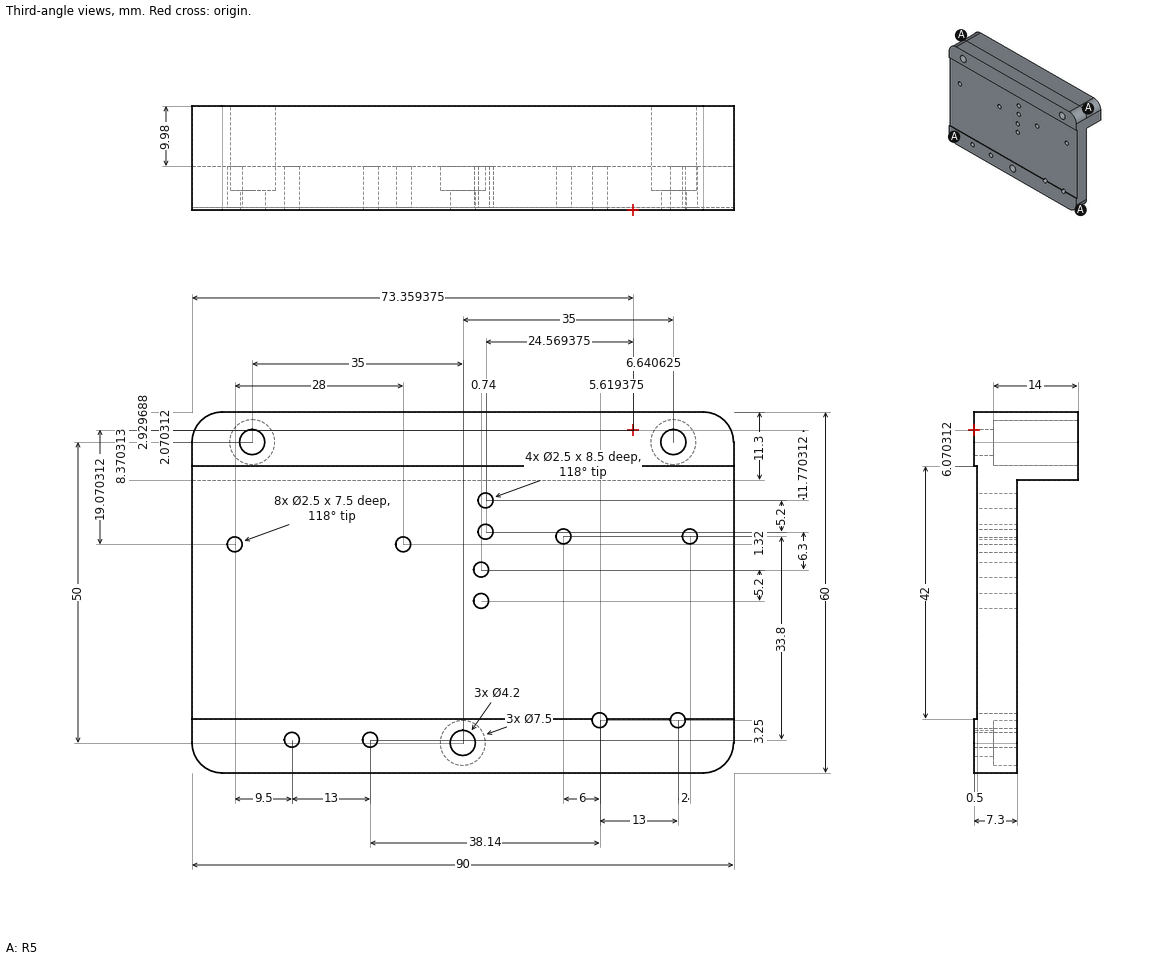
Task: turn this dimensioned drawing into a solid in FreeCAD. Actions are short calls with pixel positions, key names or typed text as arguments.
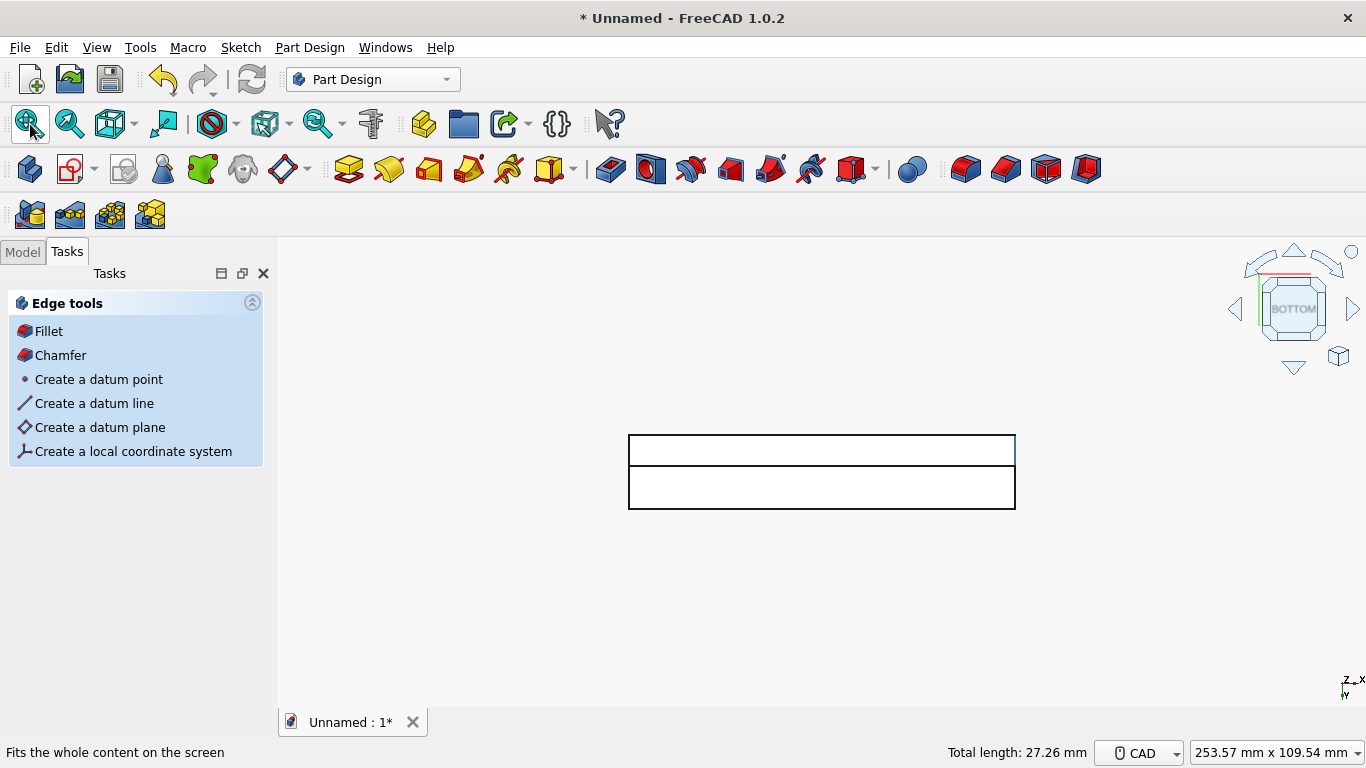
click(629, 450, ctrl)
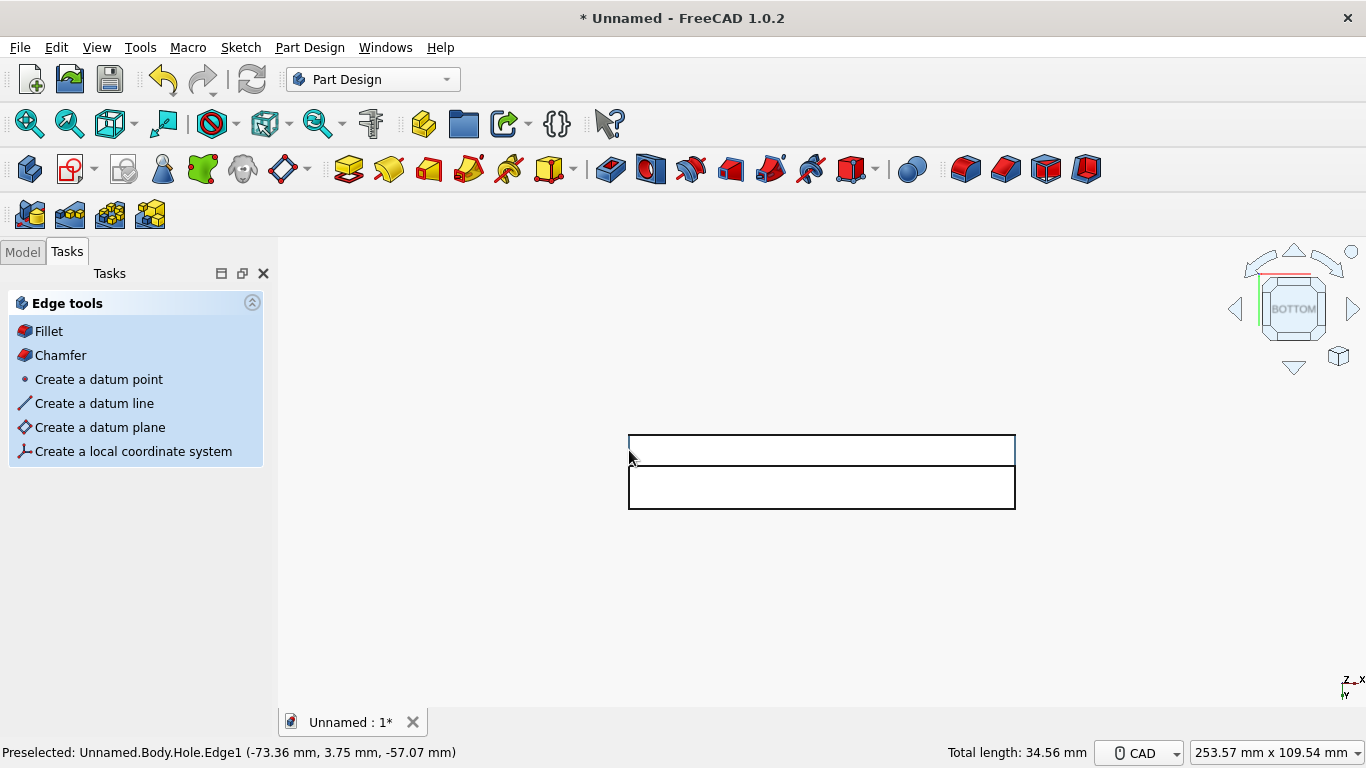
click(966, 170)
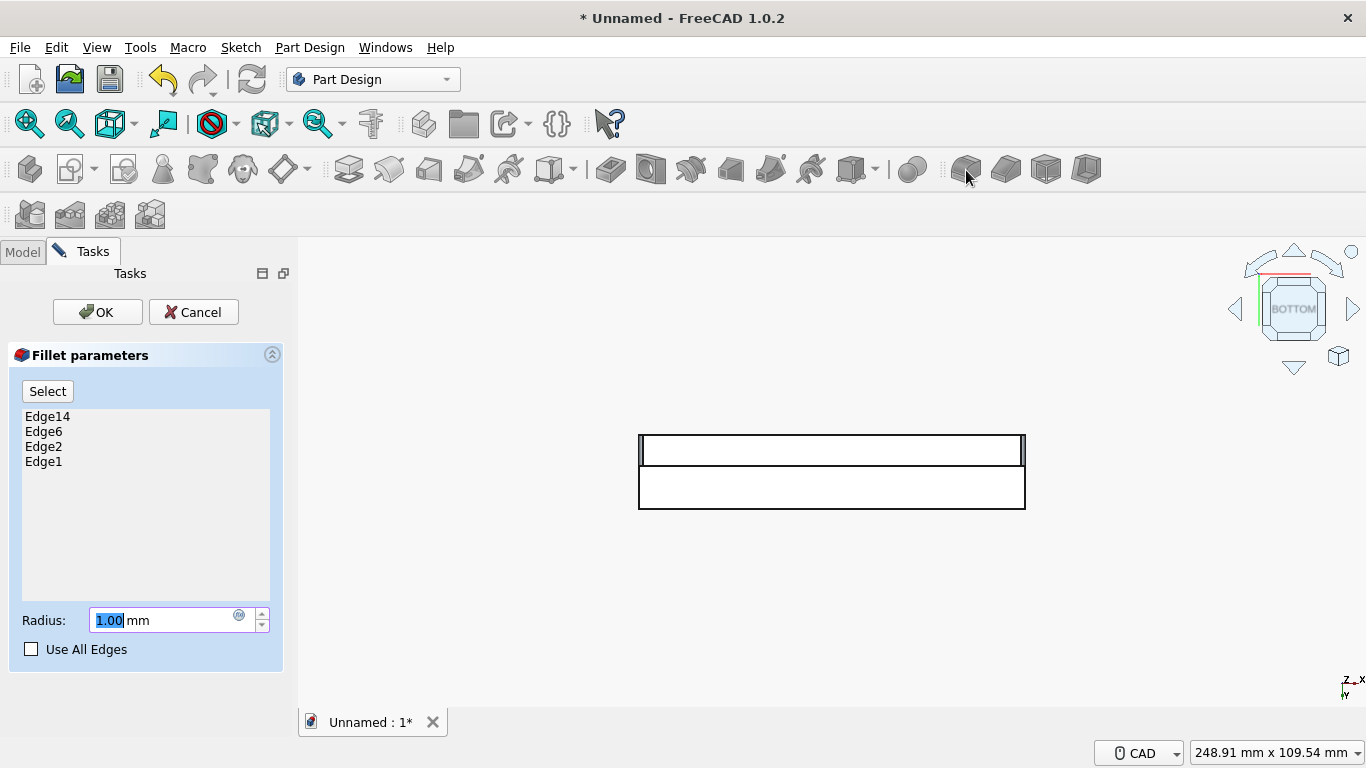
text(5)
key(Tab)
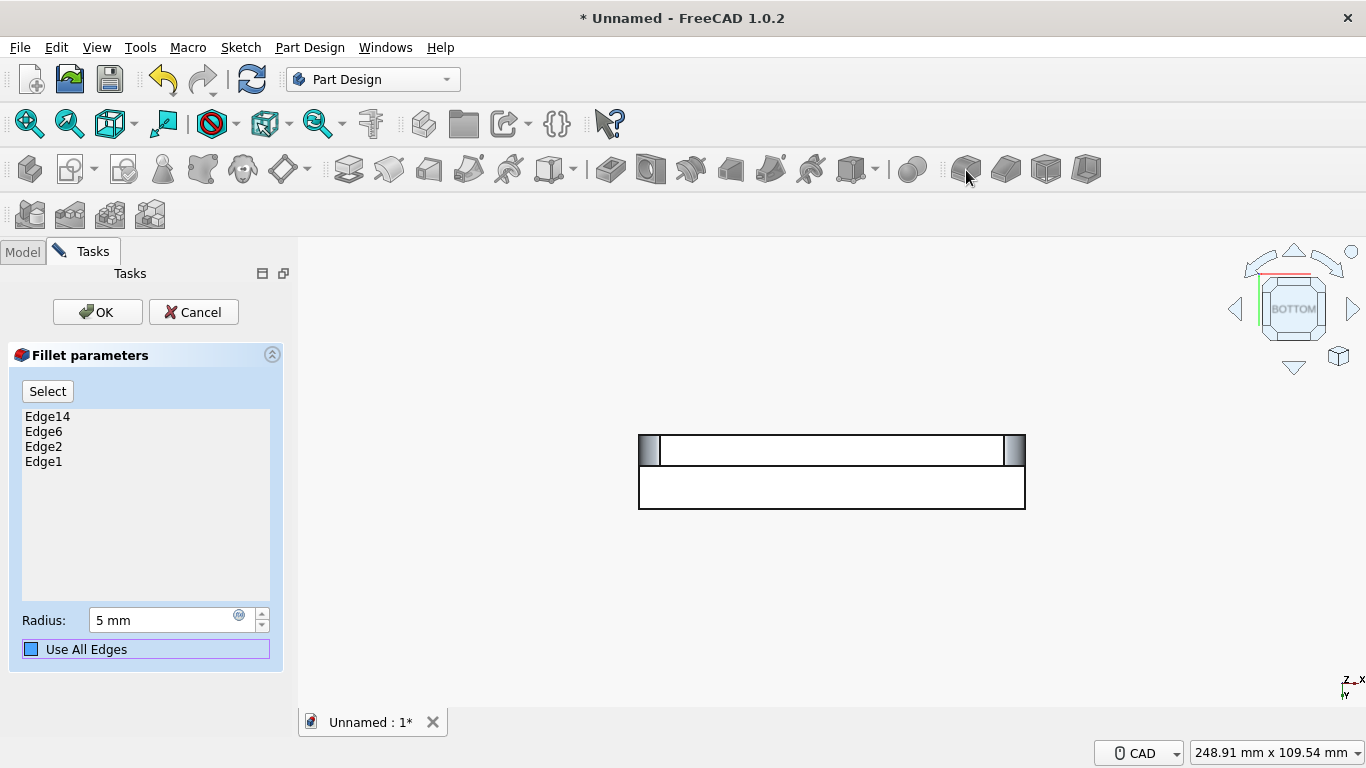
click(98, 312)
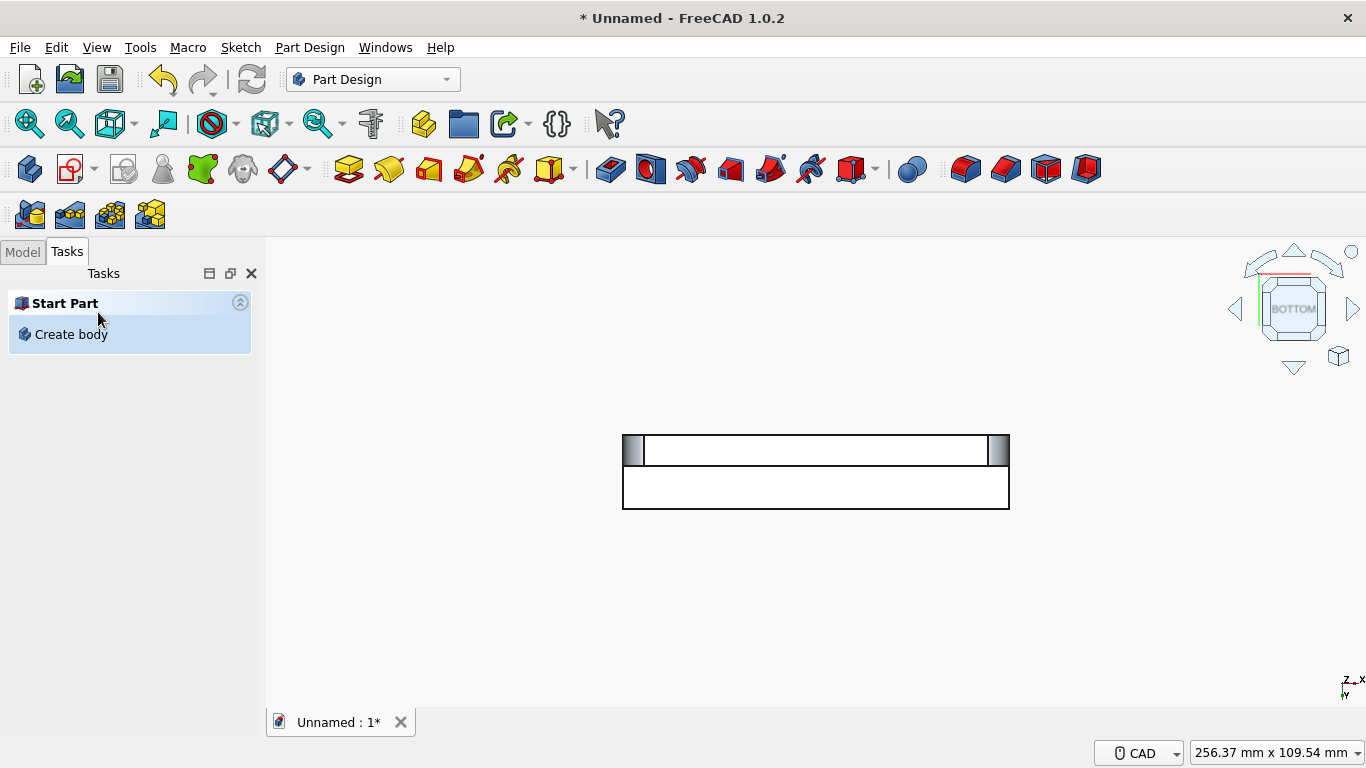
click(30, 124)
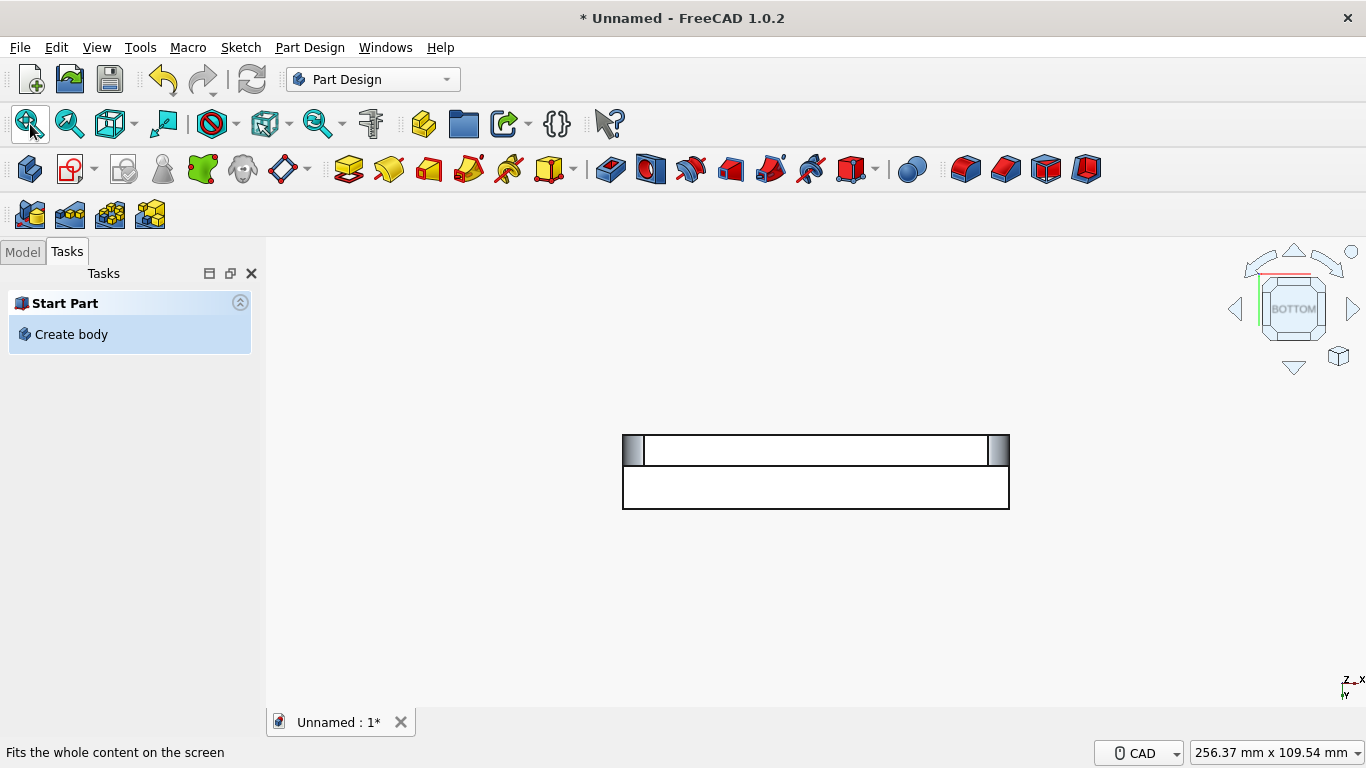
key(4)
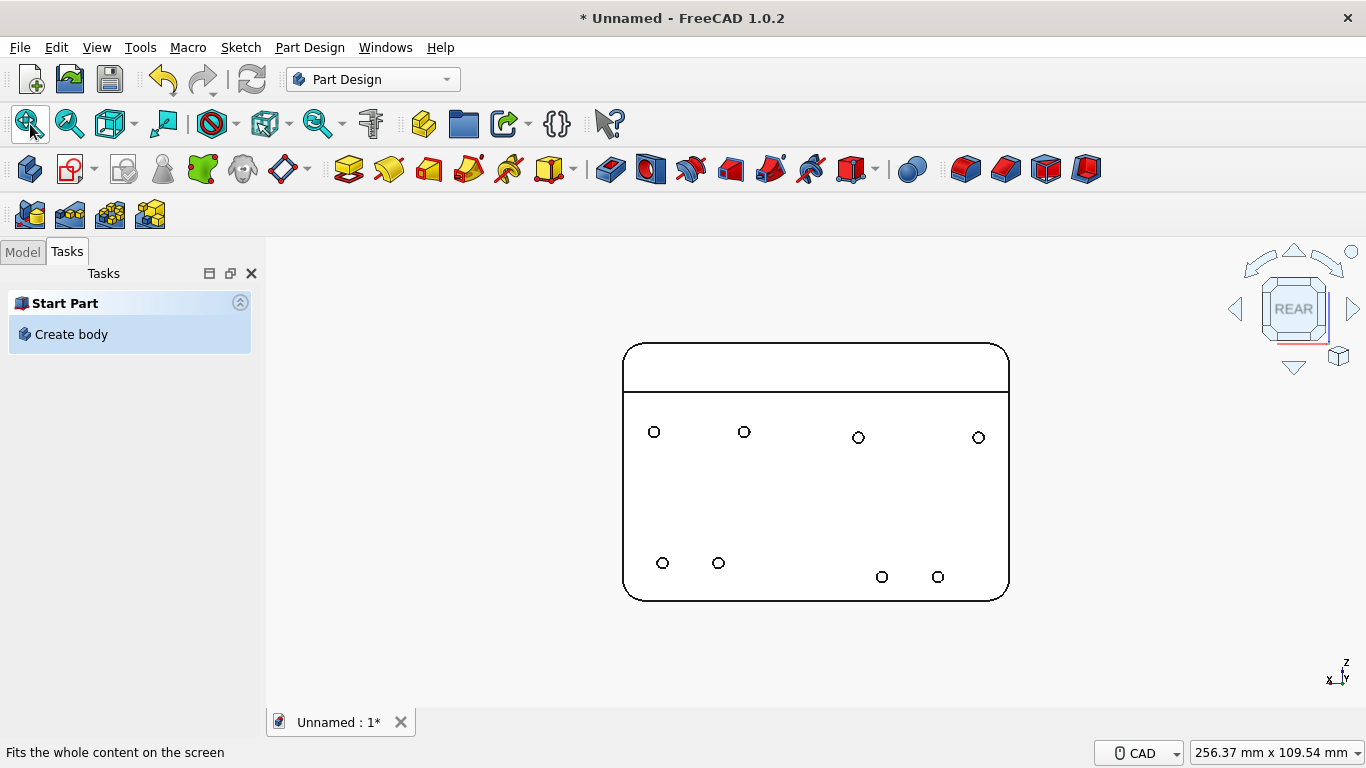
click(650, 367)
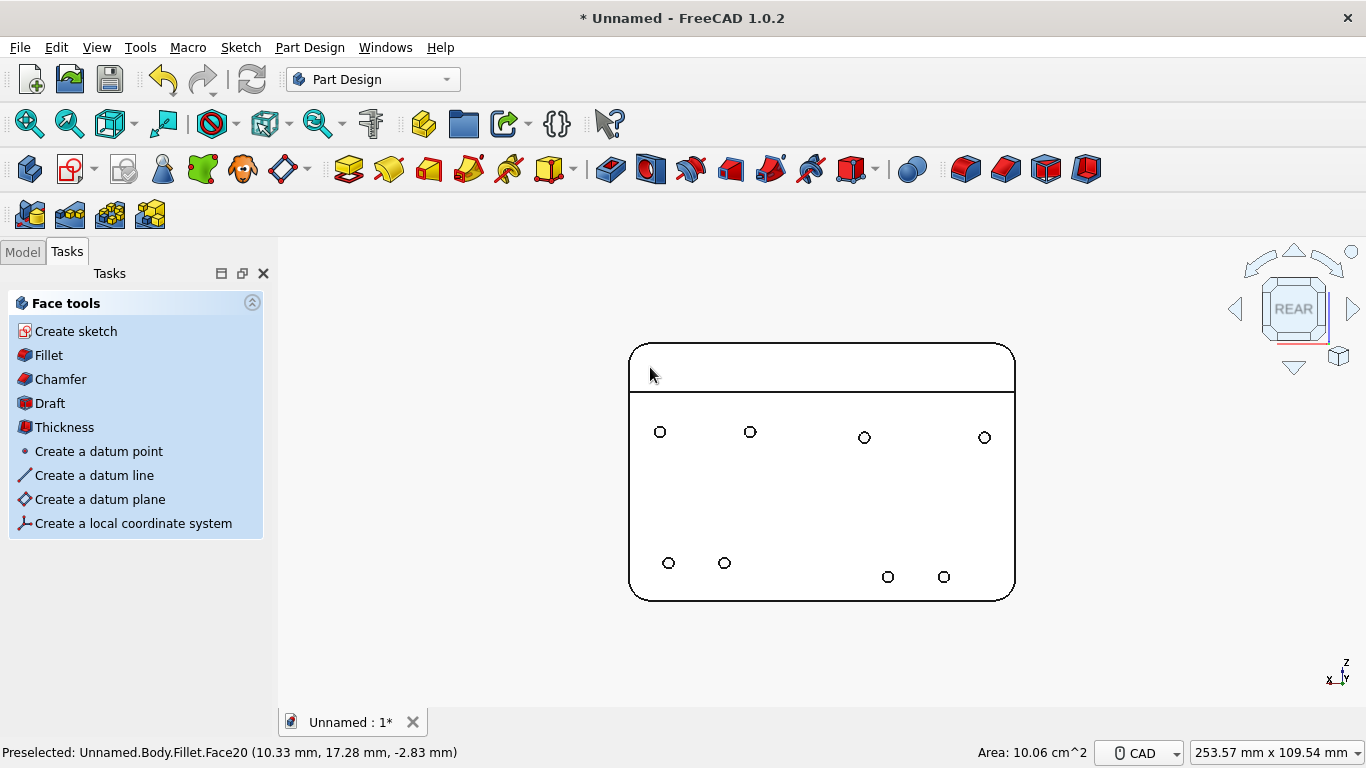
click(70, 170)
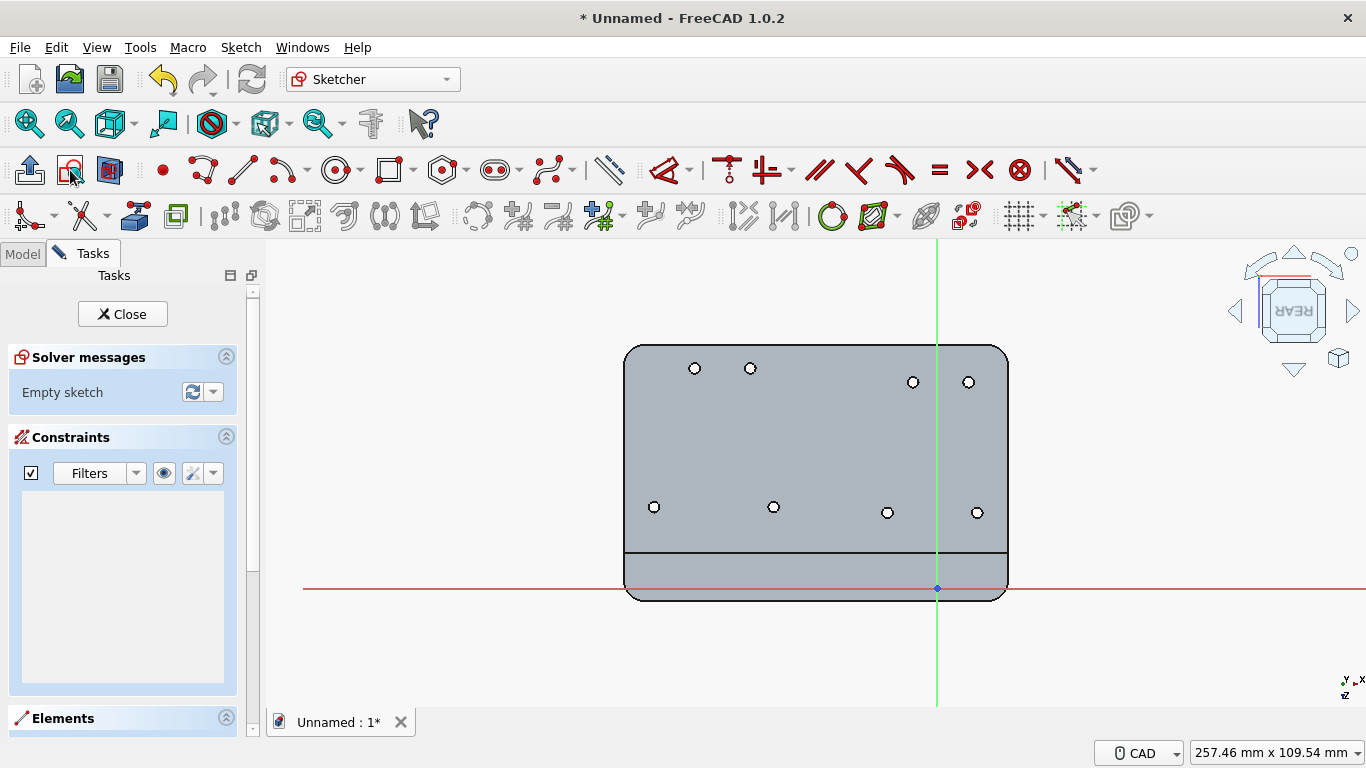
click(336, 170)